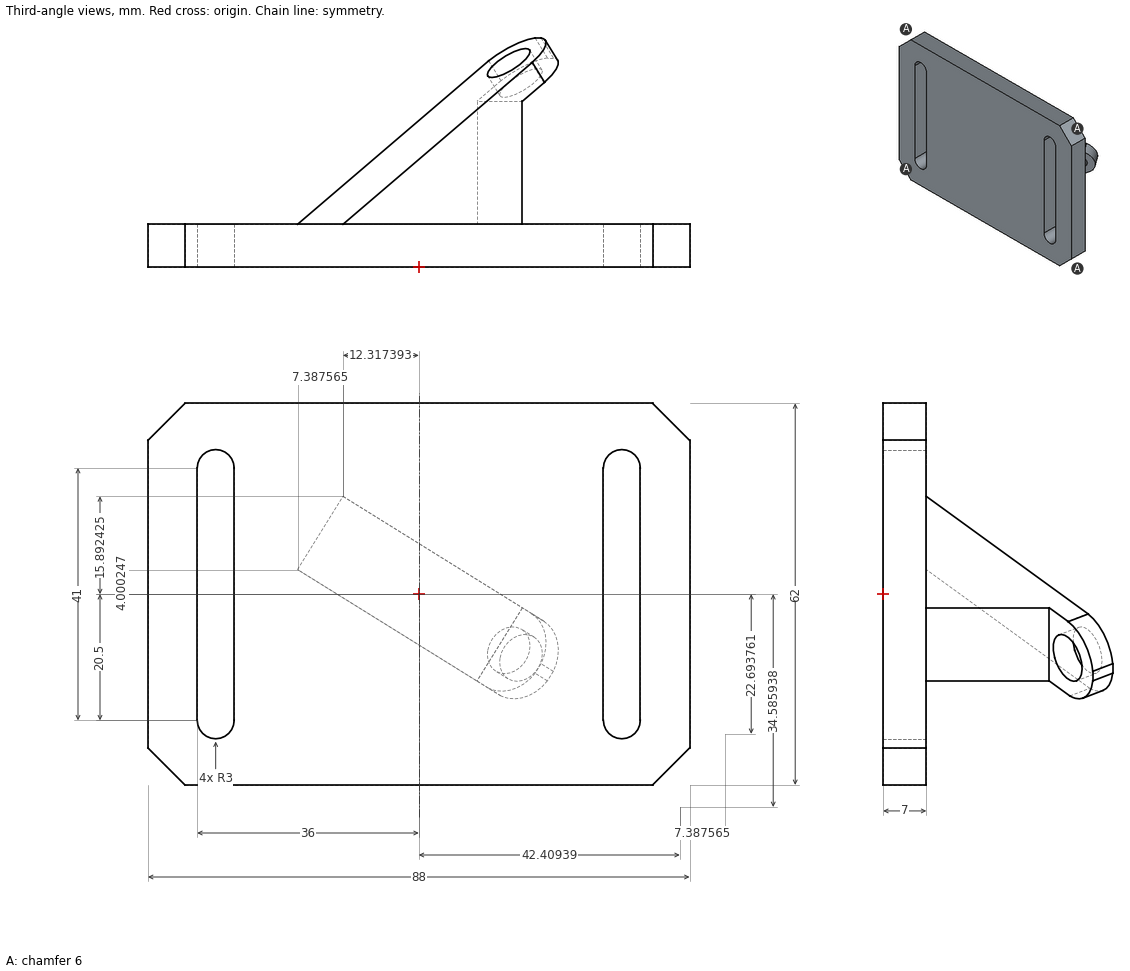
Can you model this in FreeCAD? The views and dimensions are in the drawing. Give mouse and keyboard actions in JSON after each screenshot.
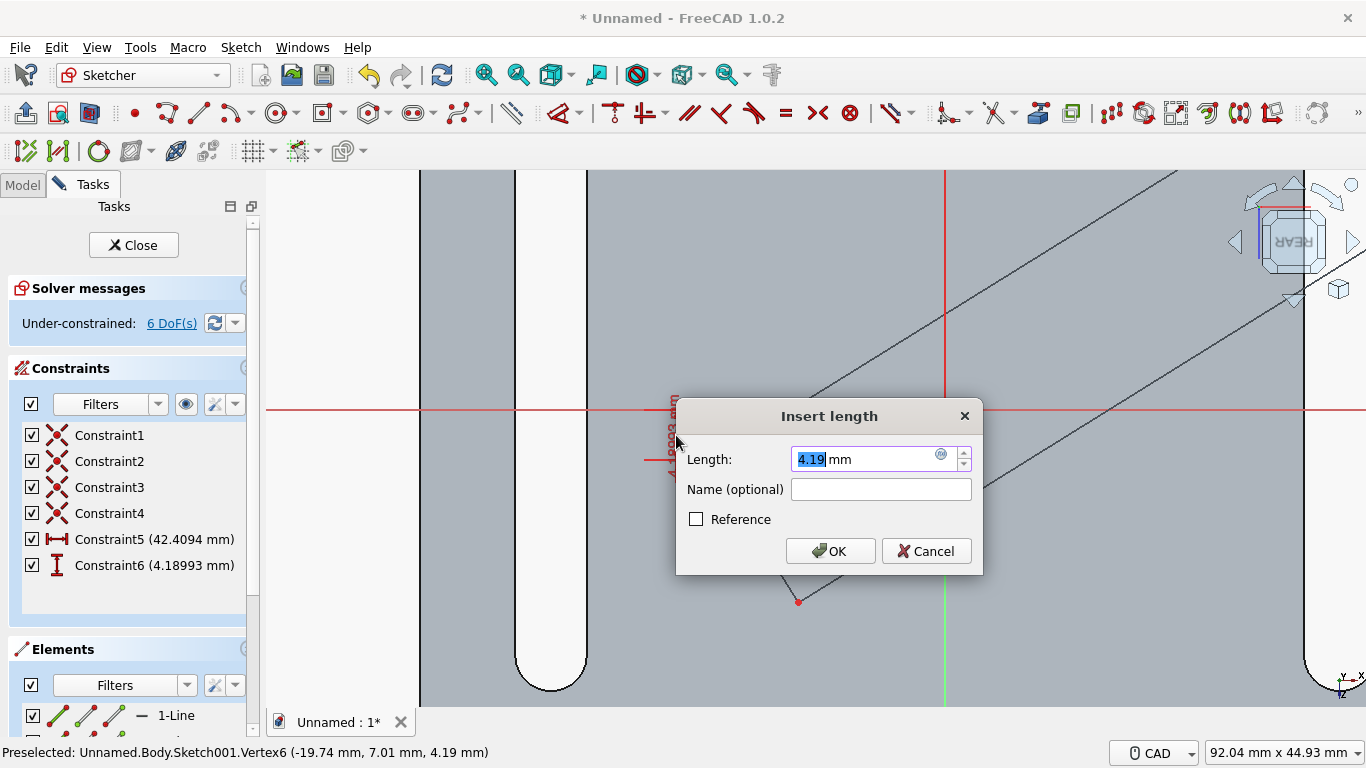
{"action": "type", "text": "4.000247"}
{"action": "key", "text": "Return"}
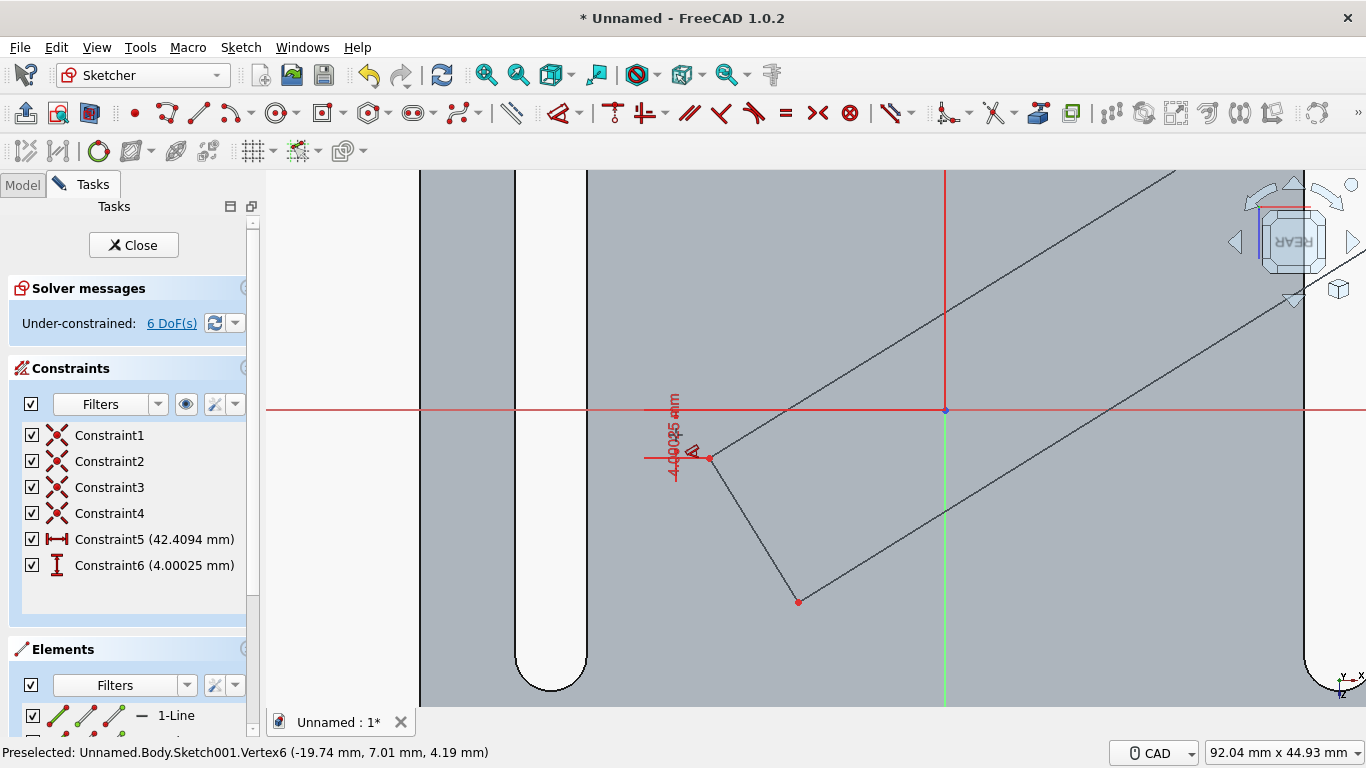
{"action": "scroll", "coordinate": [294, 609], "scroll_direction": "down", "scroll_amount": 3}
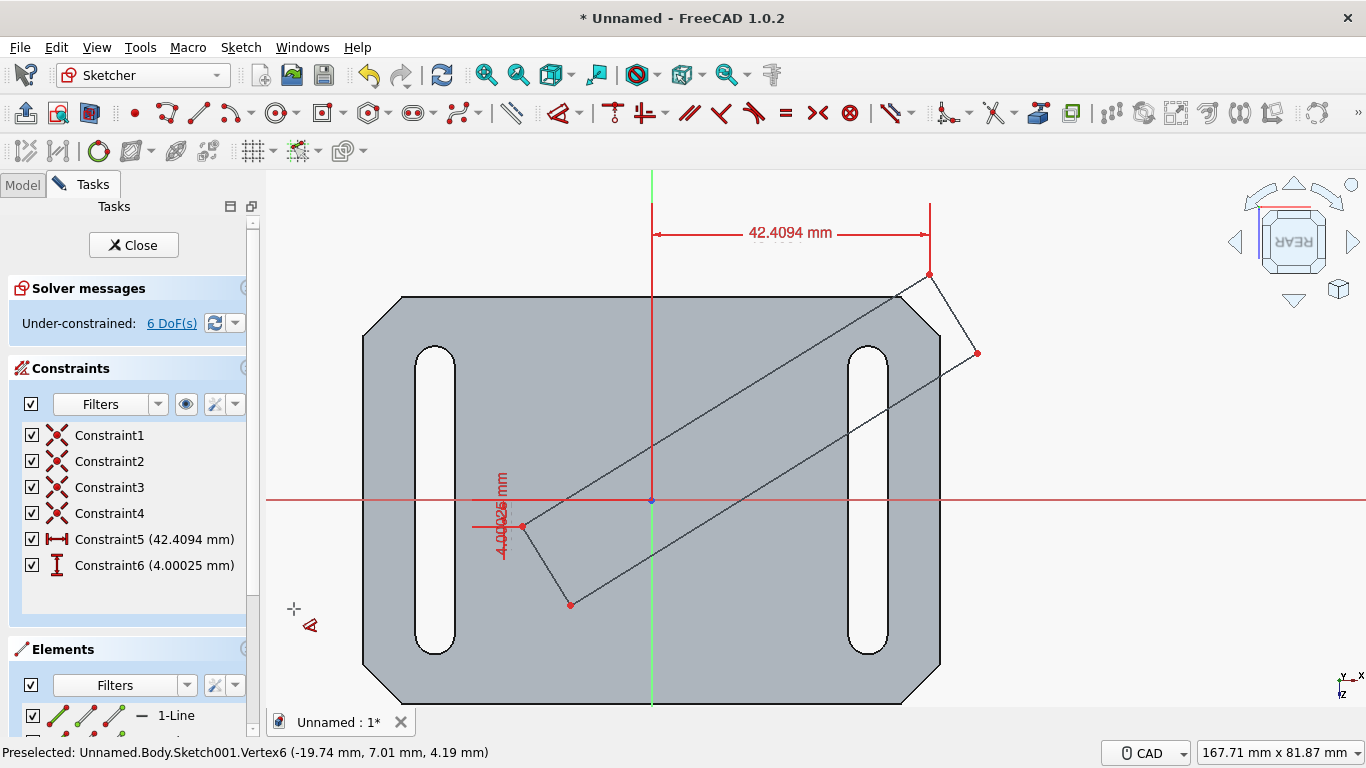
{"action": "left_click", "coordinate": [963, 330]}
{"action": "left_click", "coordinate": [954, 241]}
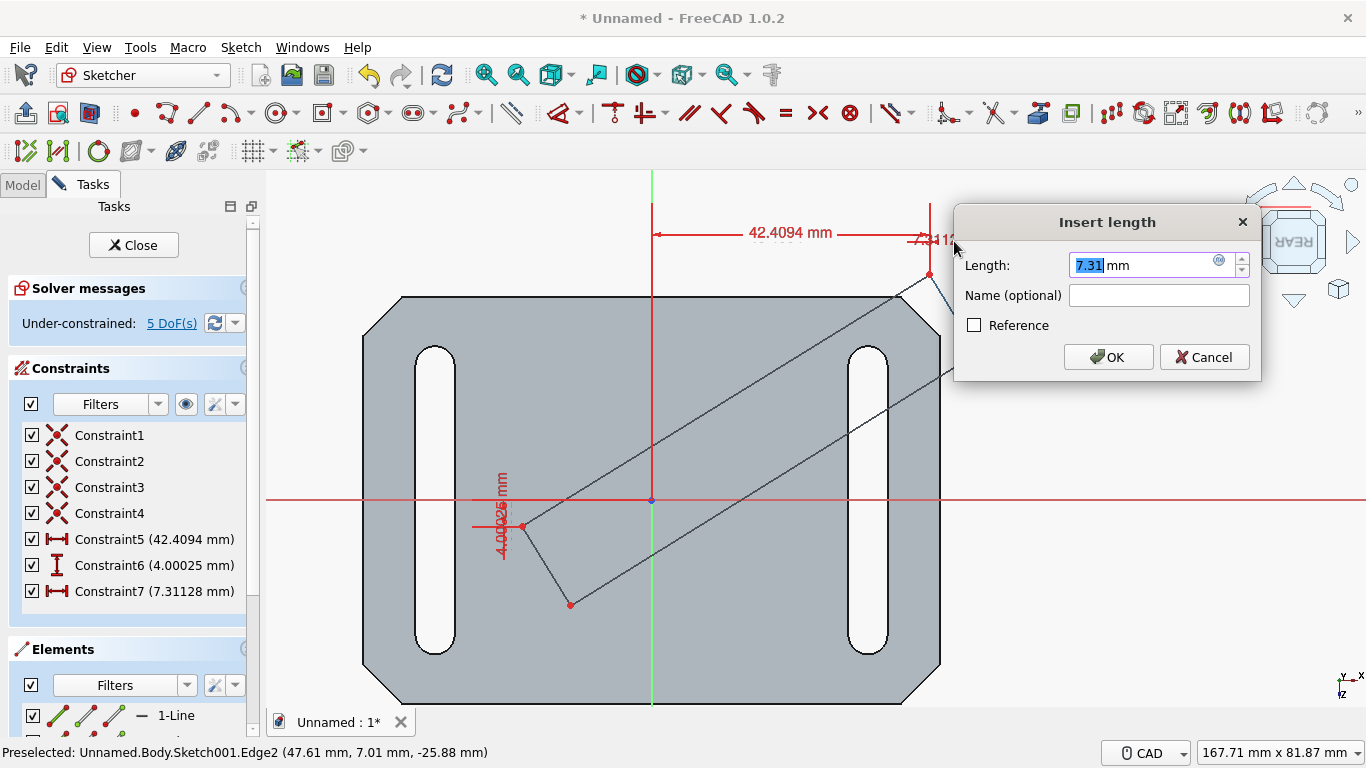
{"action": "type", "text": "7.387565"}
{"action": "key", "text": "Return"}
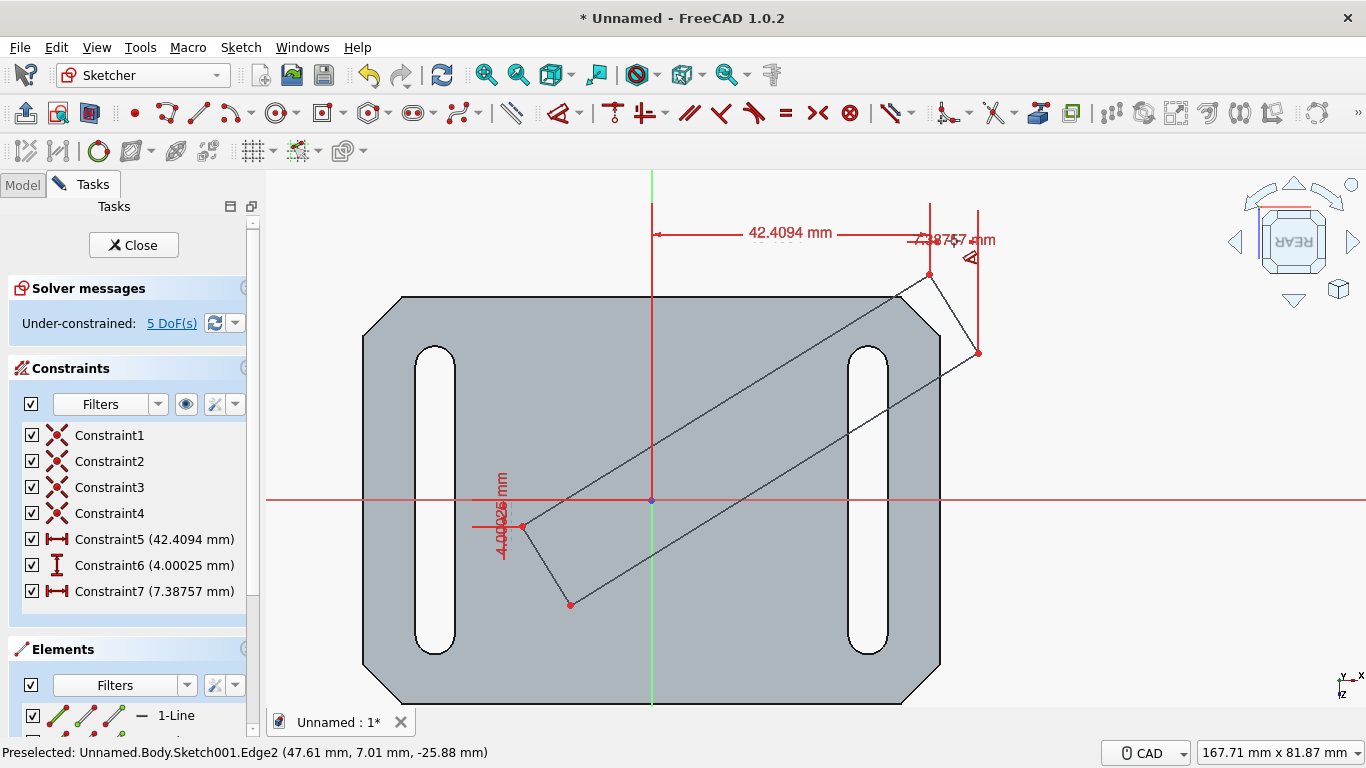
{"action": "left_click", "coordinate": [537, 550]}
{"action": "left_click", "coordinate": [546, 640]}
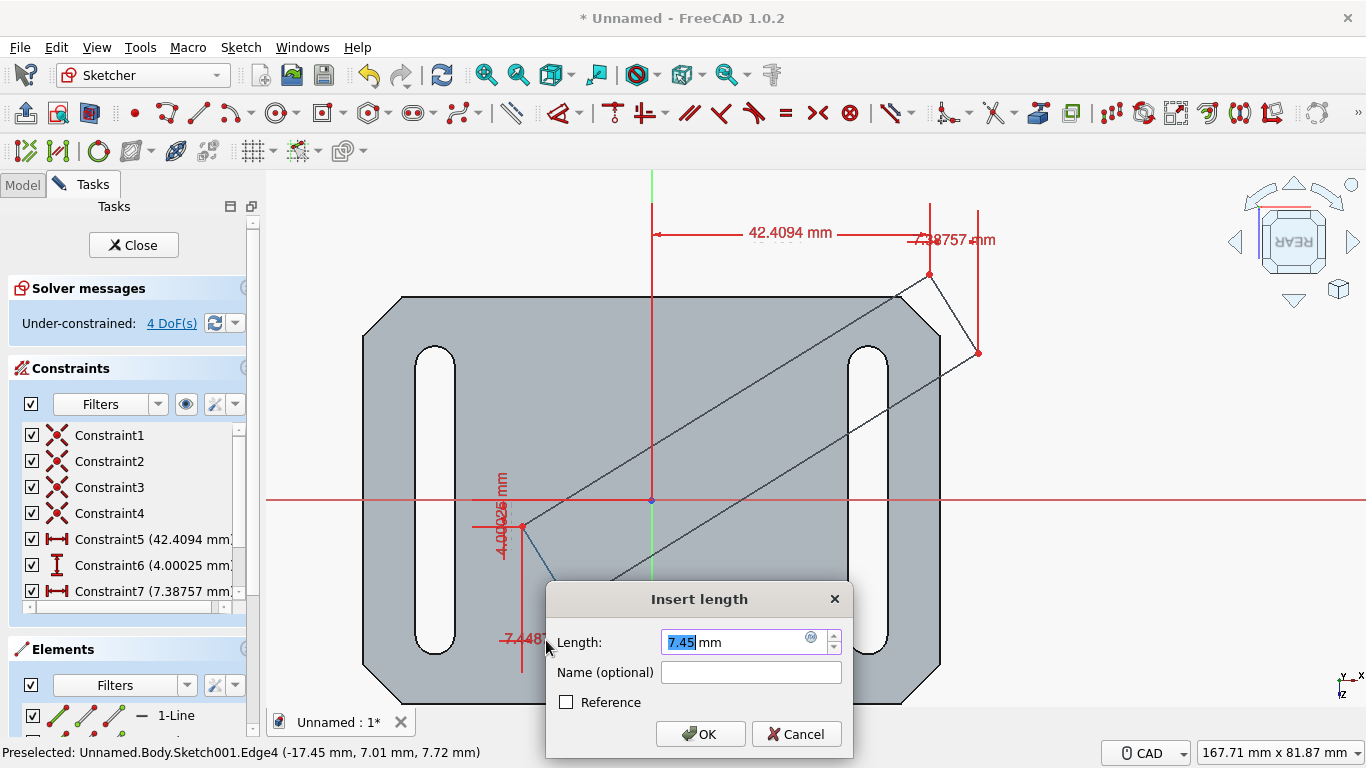
{"action": "type", "text": "7.387565"}
{"action": "key", "text": "Return"}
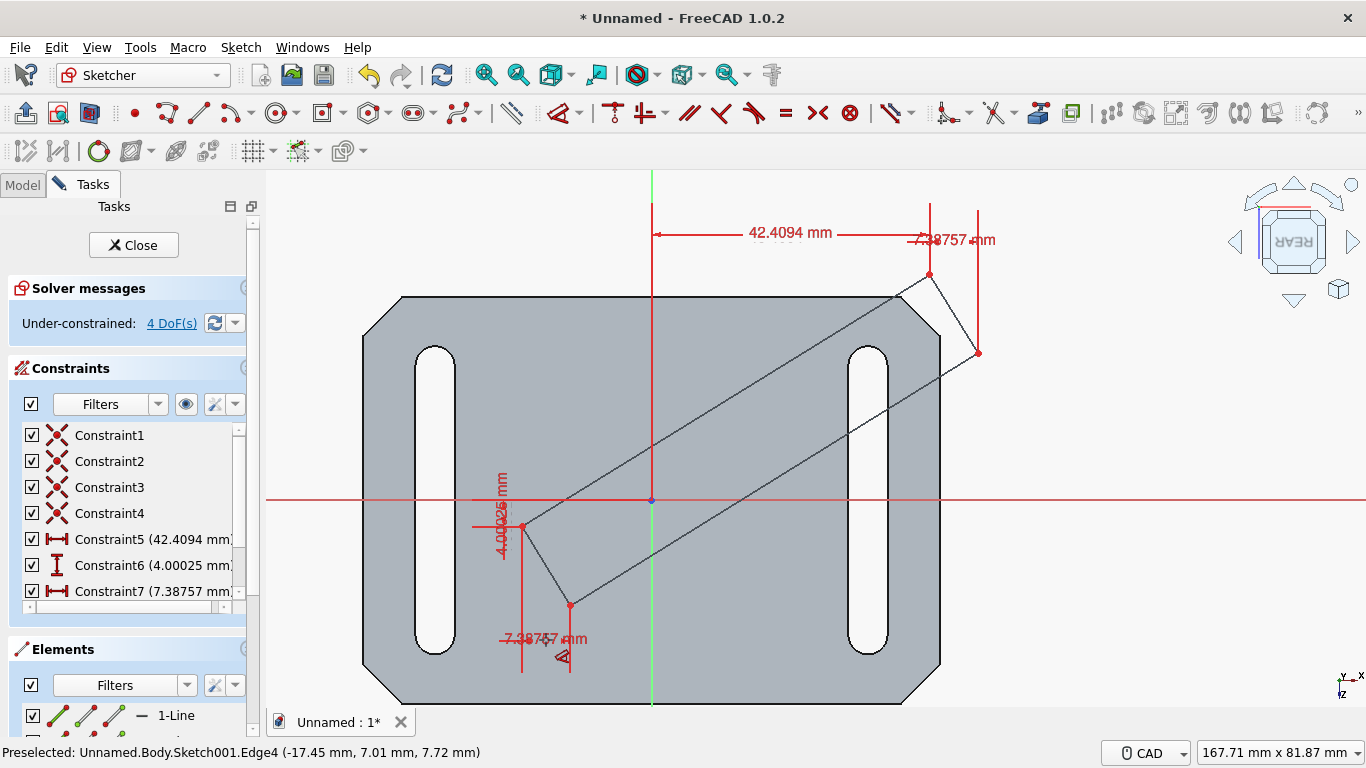
{"action": "left_click", "coordinate": [570, 606]}
{"action": "left_click", "coordinate": [630, 640]}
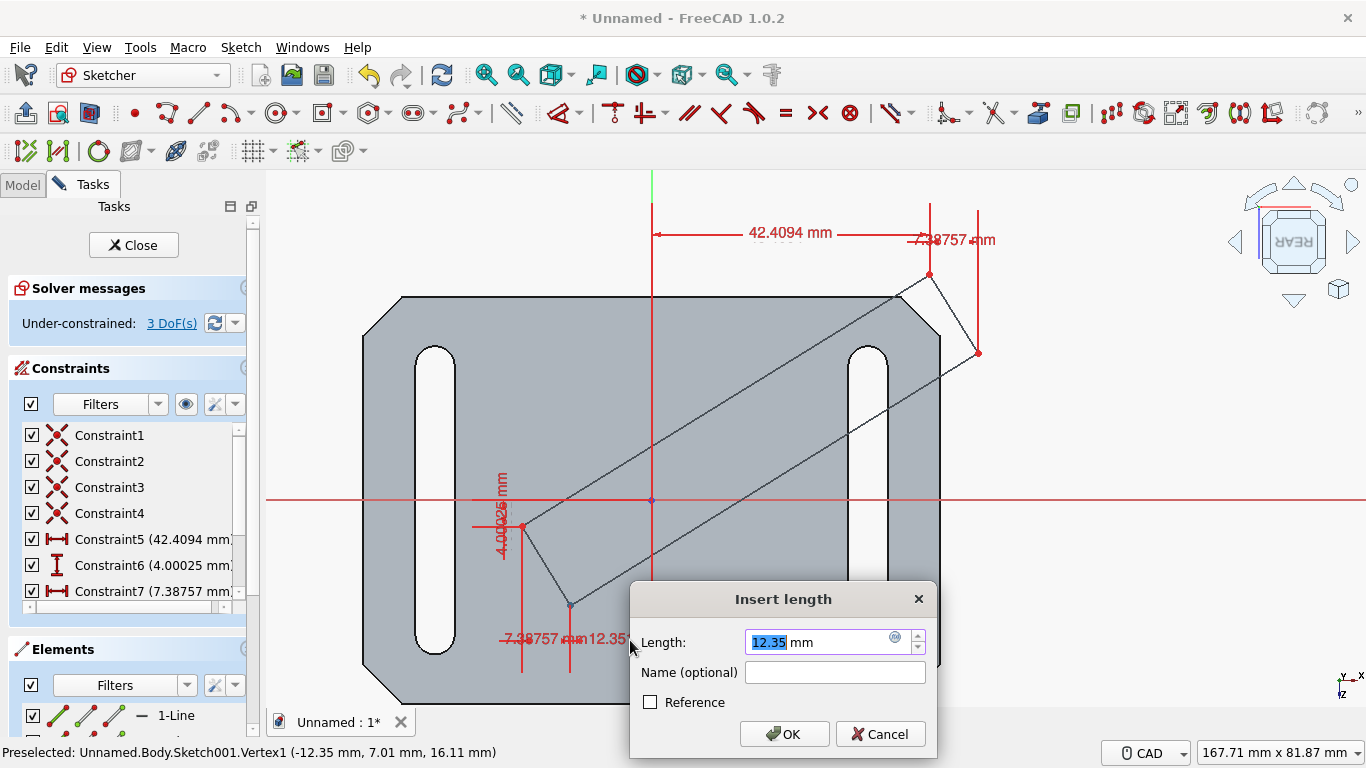
{"action": "type", "text": "12.317393"}
{"action": "key", "text": "Return"}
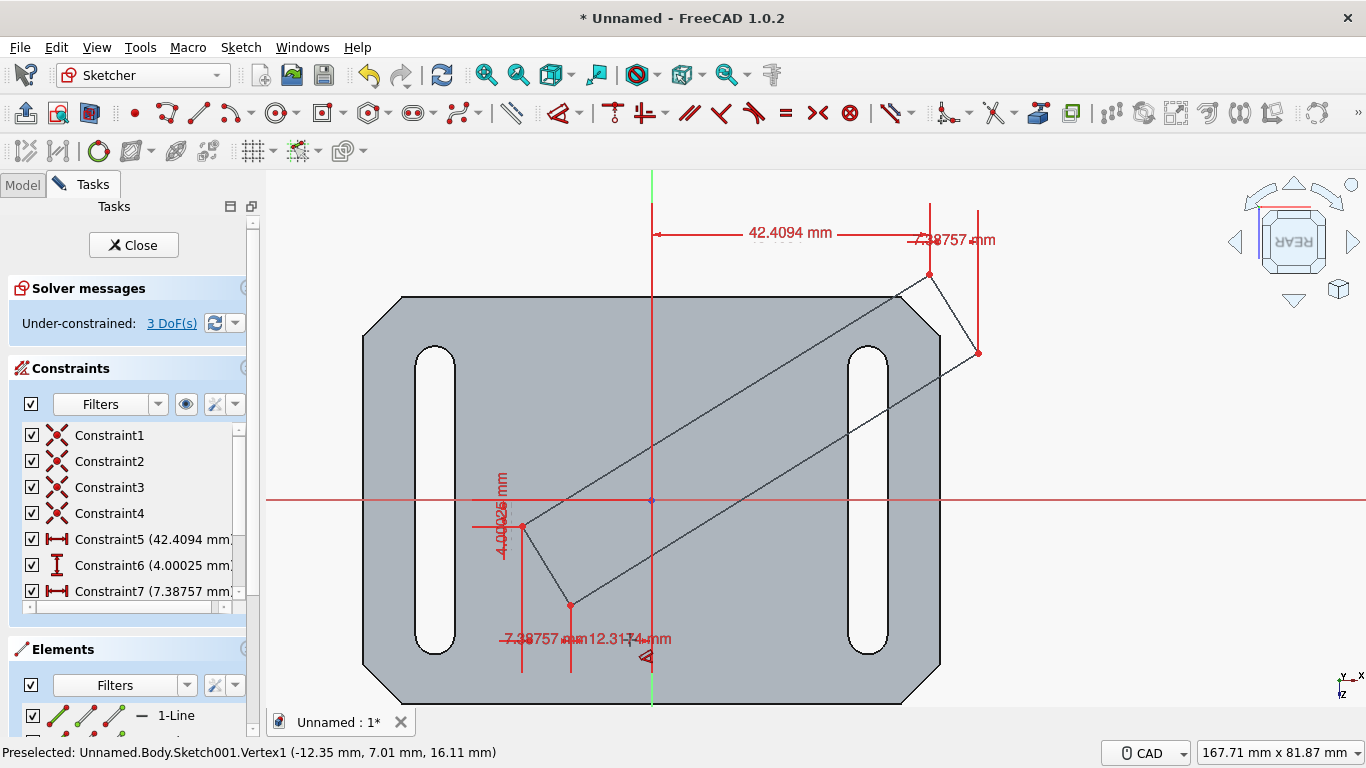
{"action": "left_click", "coordinate": [571, 606]}
{"action": "left_click", "coordinate": [537, 577]}